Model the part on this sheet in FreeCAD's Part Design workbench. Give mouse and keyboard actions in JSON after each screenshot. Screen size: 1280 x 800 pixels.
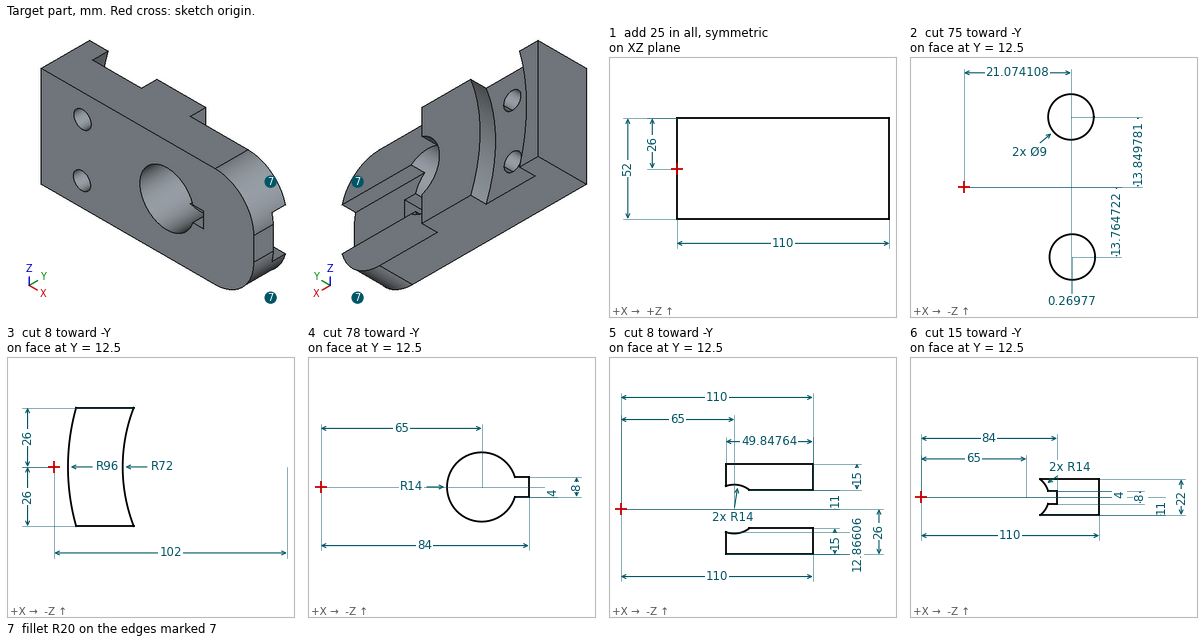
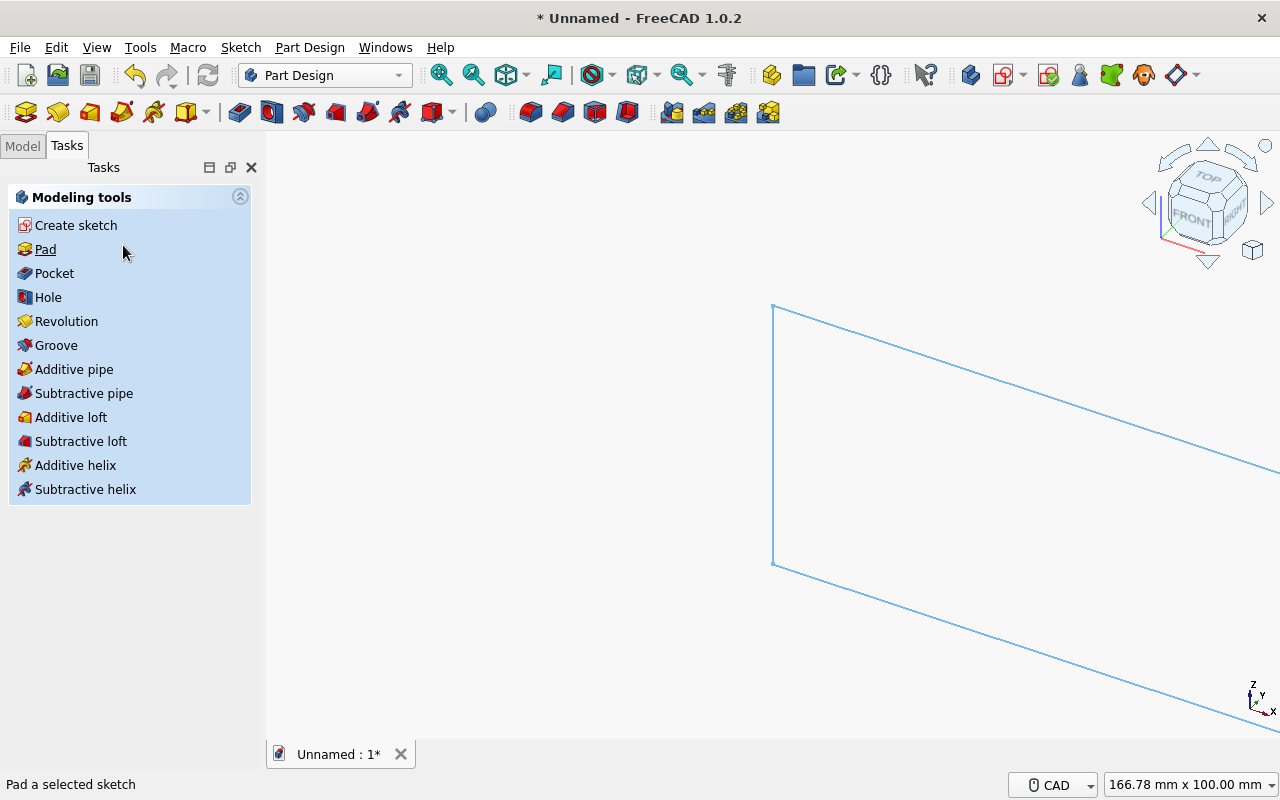
{"action": "left_click", "coordinate": [26, 112]}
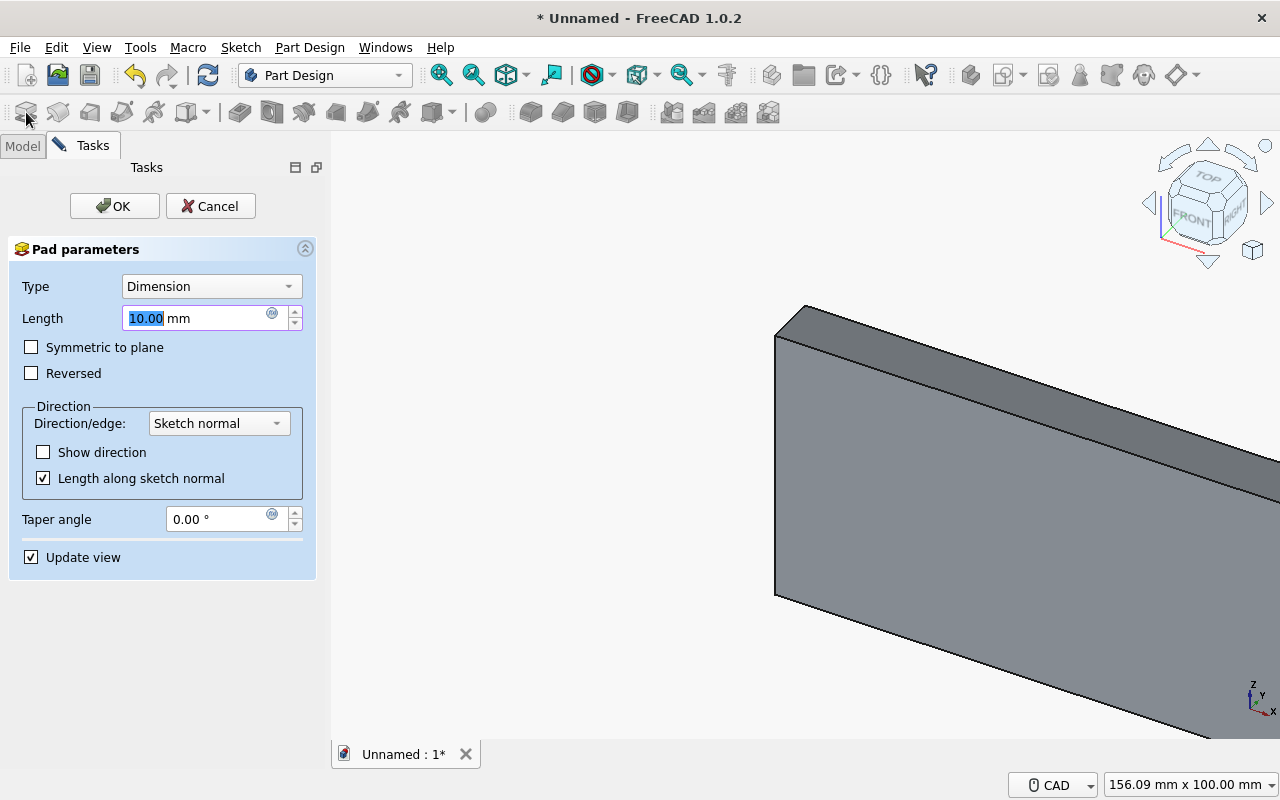
{"action": "type", "text": "25"}
{"action": "key", "text": "Tab"}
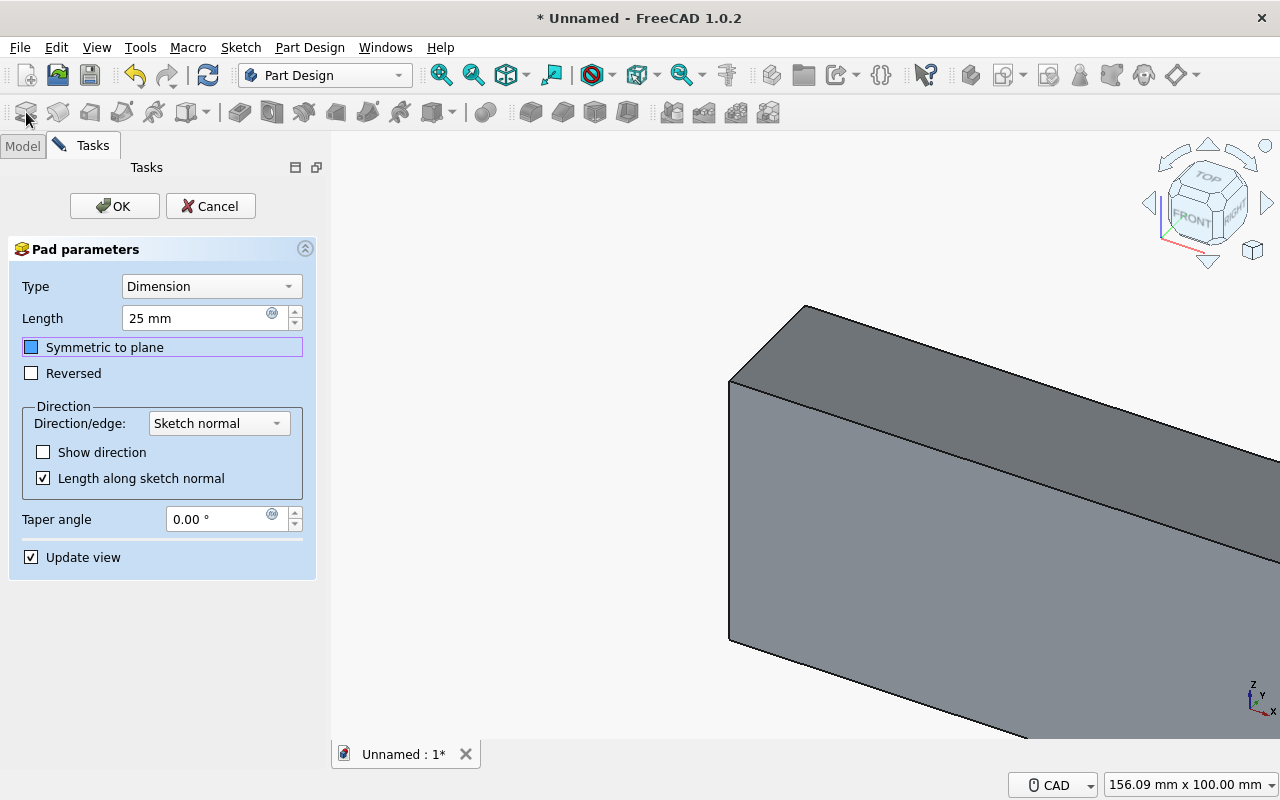
{"action": "left_click", "coordinate": [30, 347]}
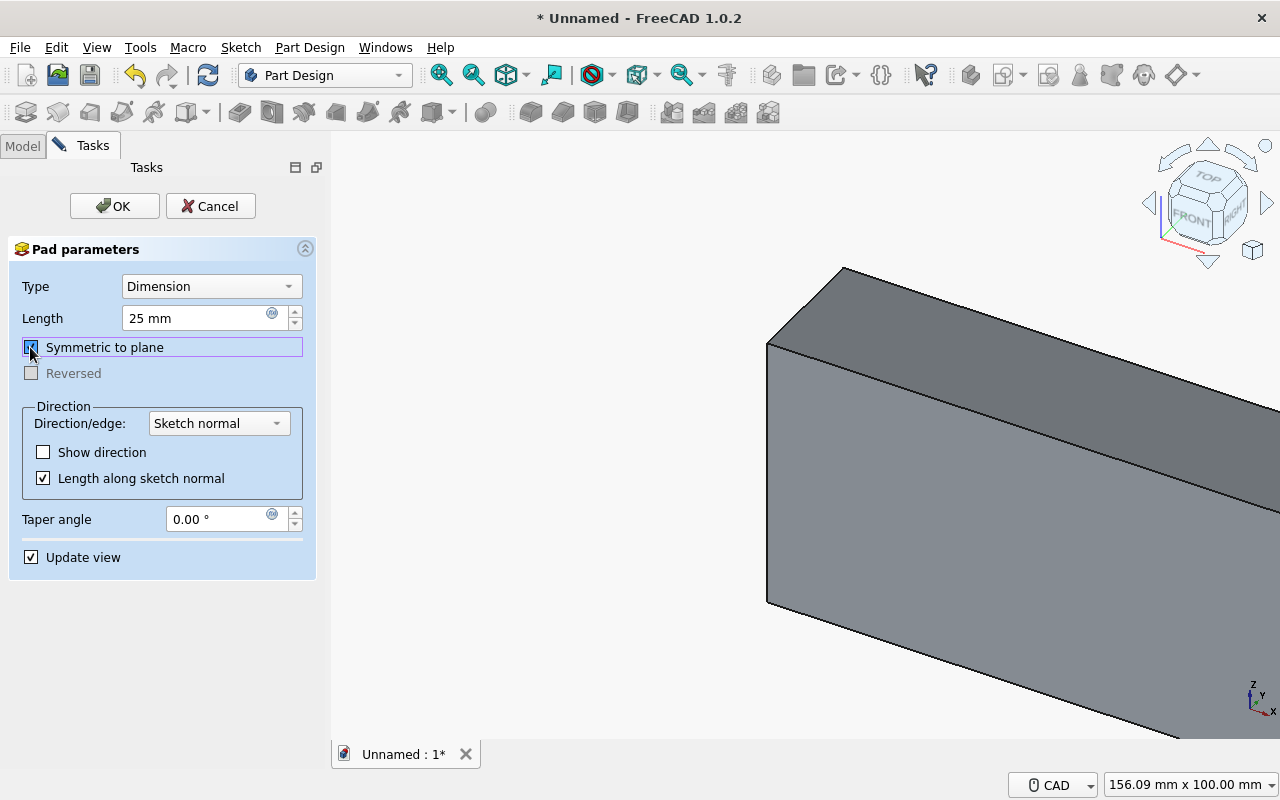
{"action": "left_click", "coordinate": [115, 206]}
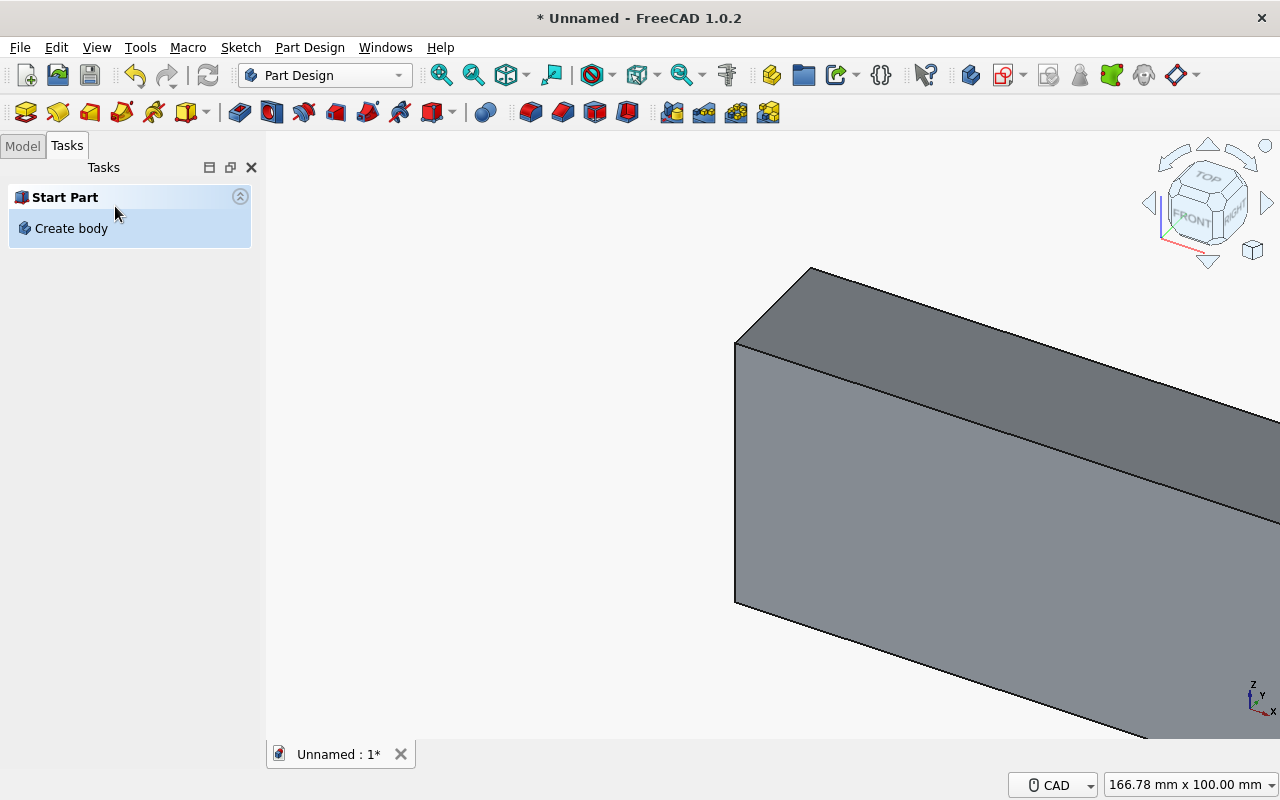
{"action": "left_click", "coordinate": [442, 76]}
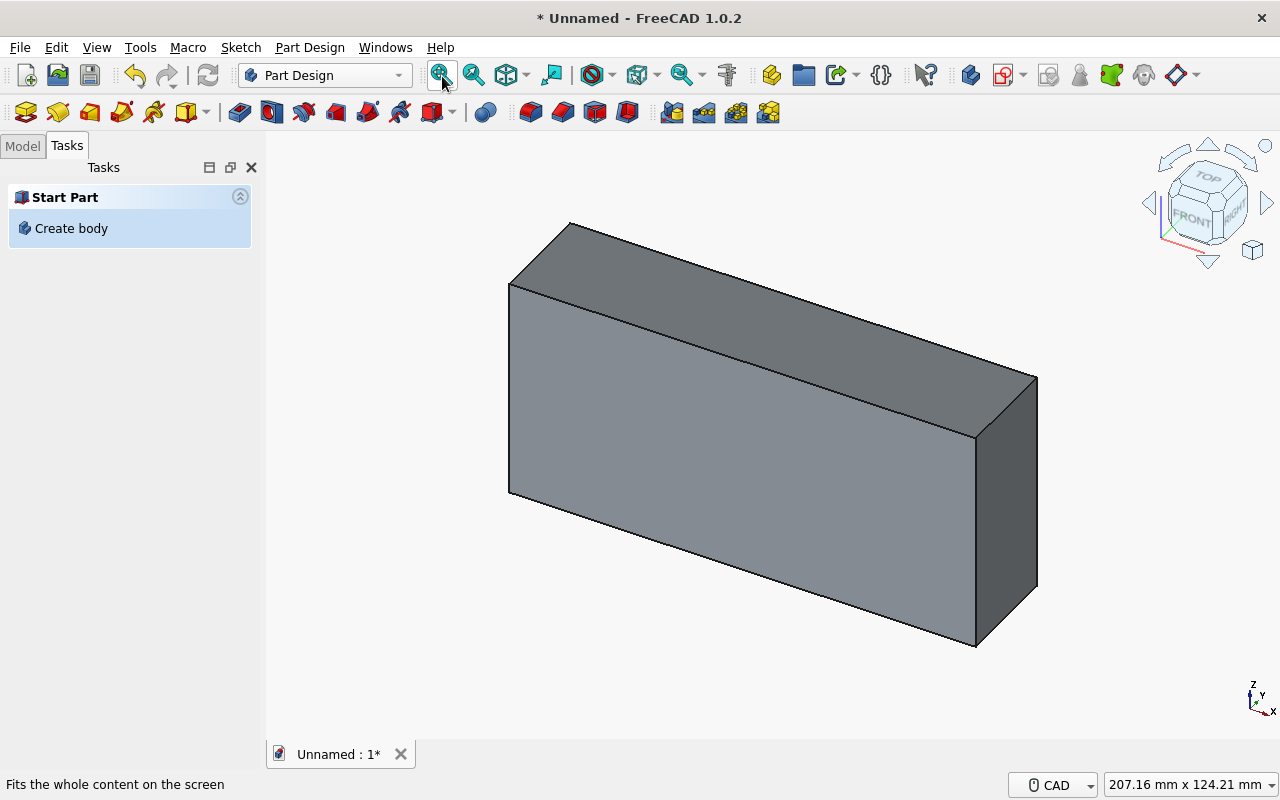
{"action": "key", "text": "4"}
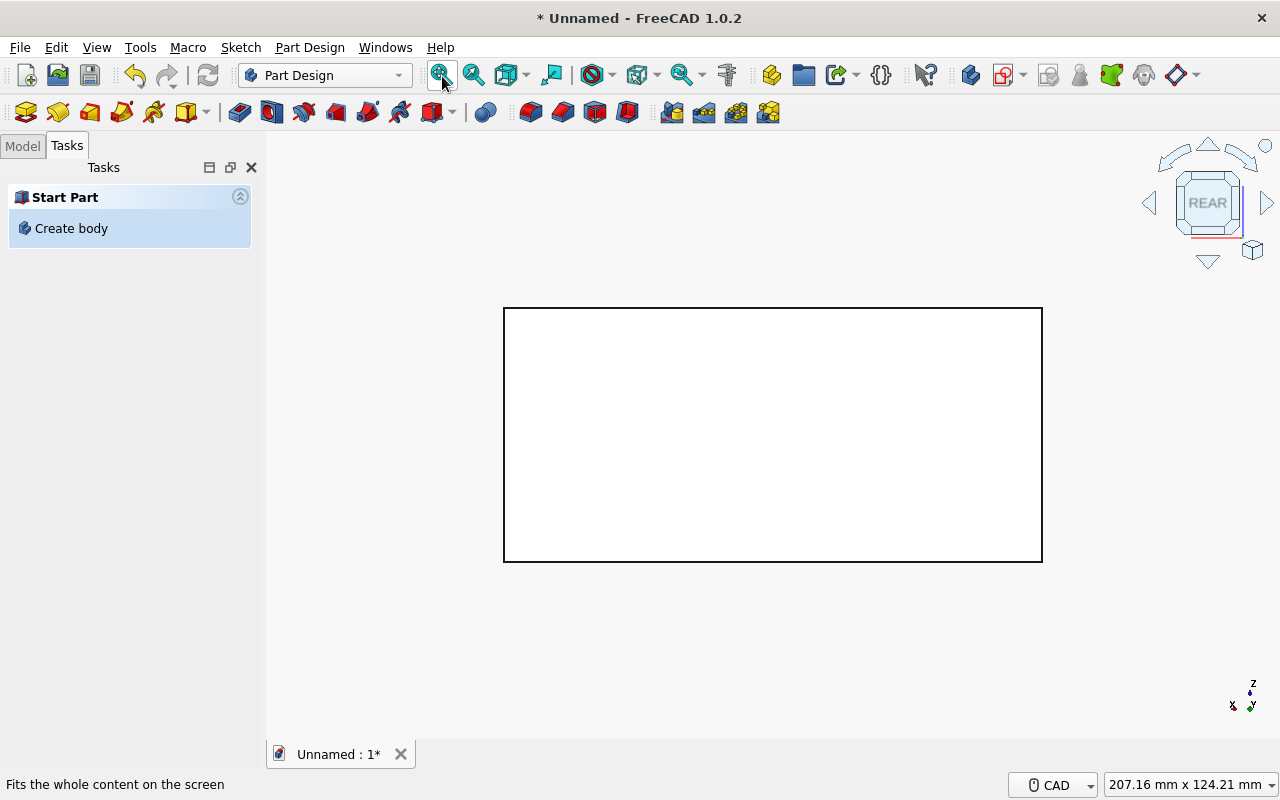
{"action": "left_click", "coordinate": [696, 434]}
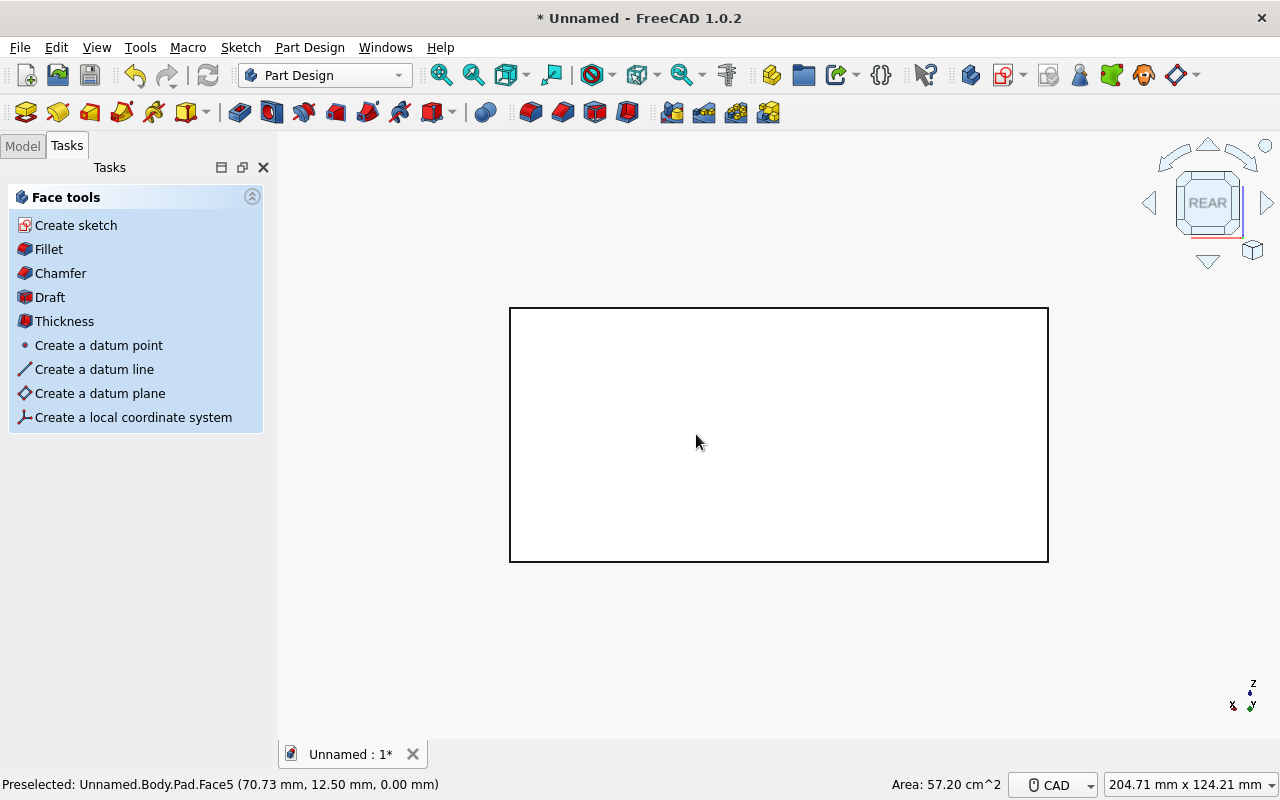
{"action": "left_click", "coordinate": [1004, 76]}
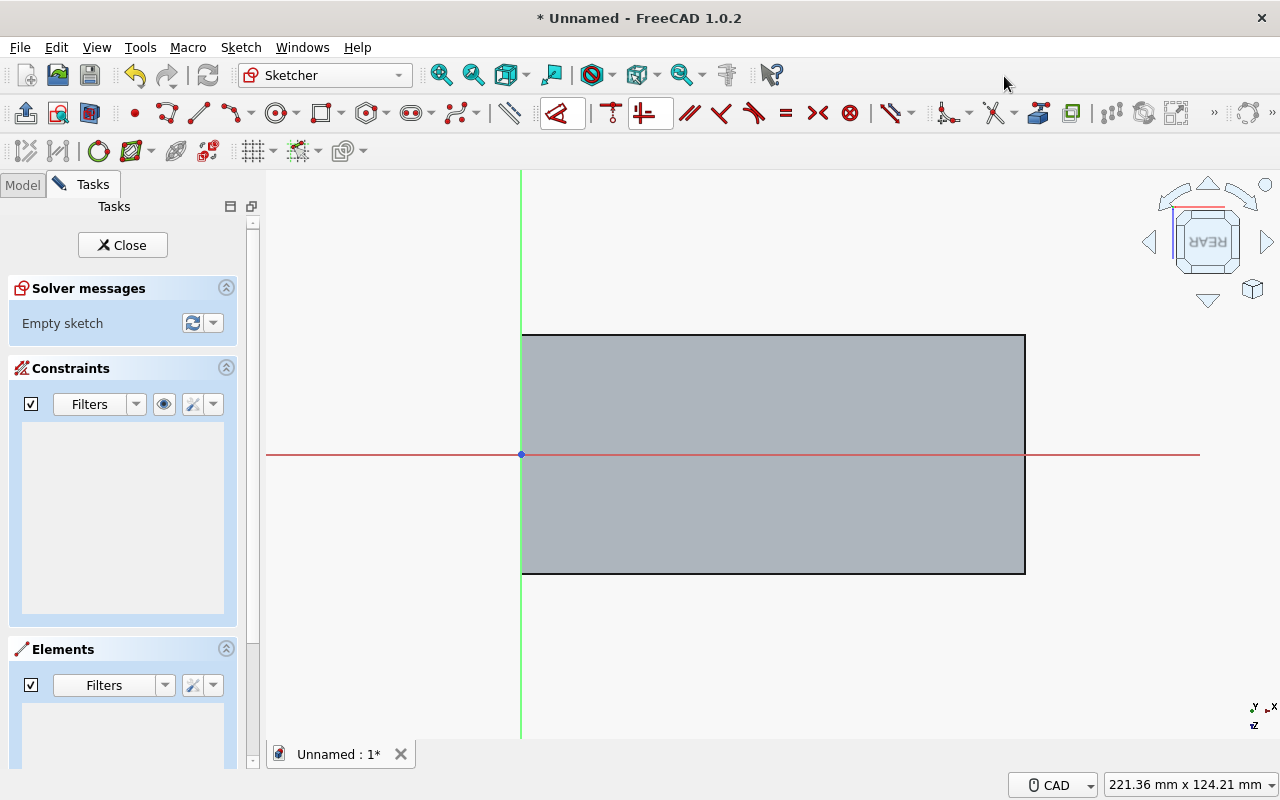
{"action": "scroll", "coordinate": [479, 454], "scroll_direction": "up", "scroll_amount": 4}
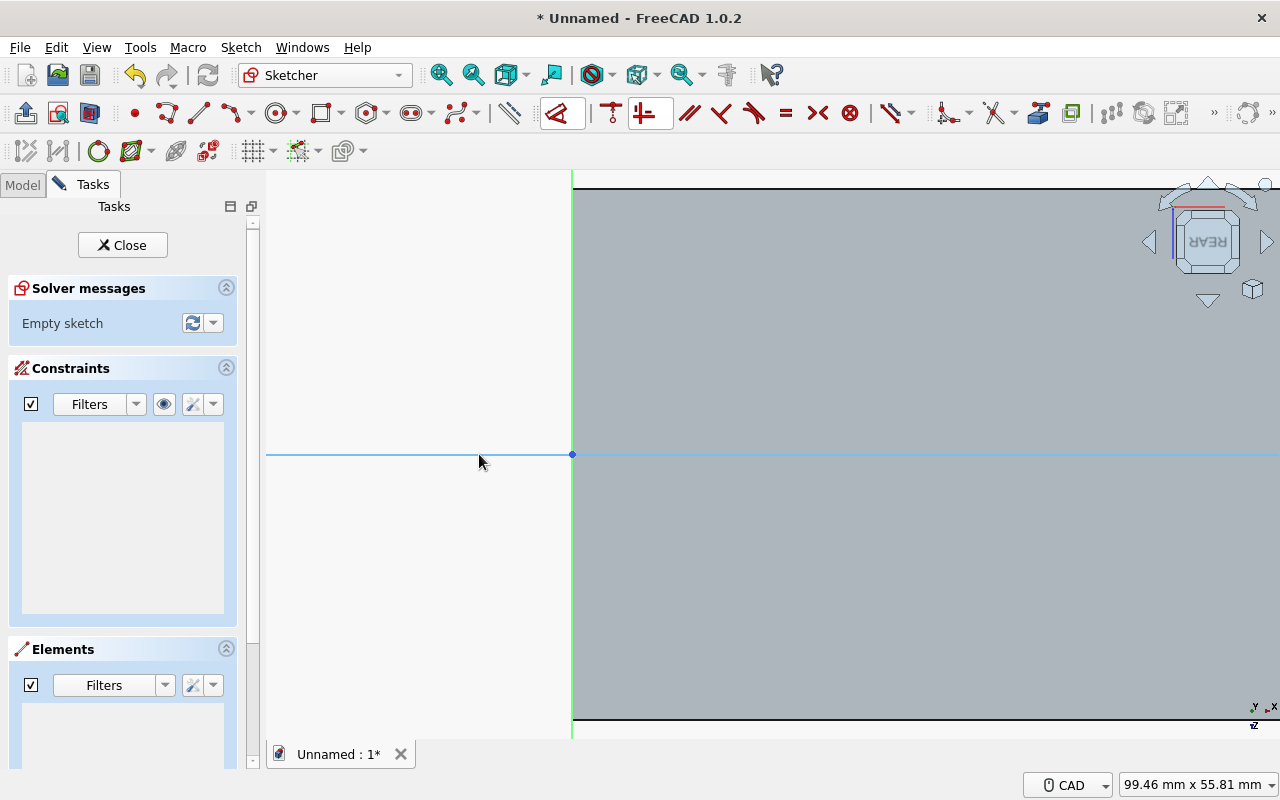
{"action": "left_click", "coordinate": [276, 114]}